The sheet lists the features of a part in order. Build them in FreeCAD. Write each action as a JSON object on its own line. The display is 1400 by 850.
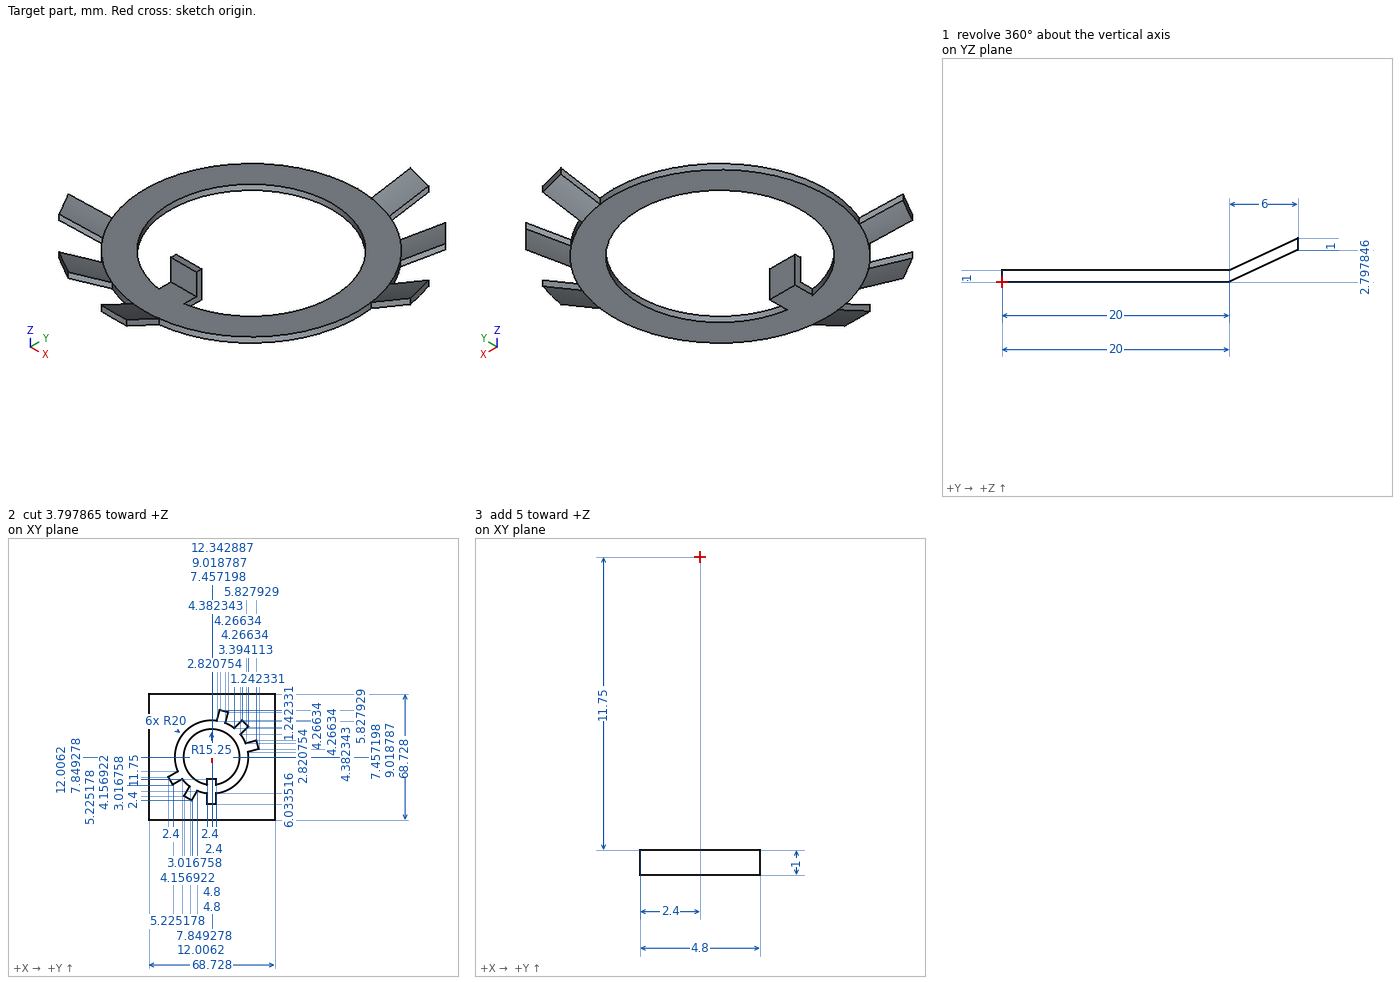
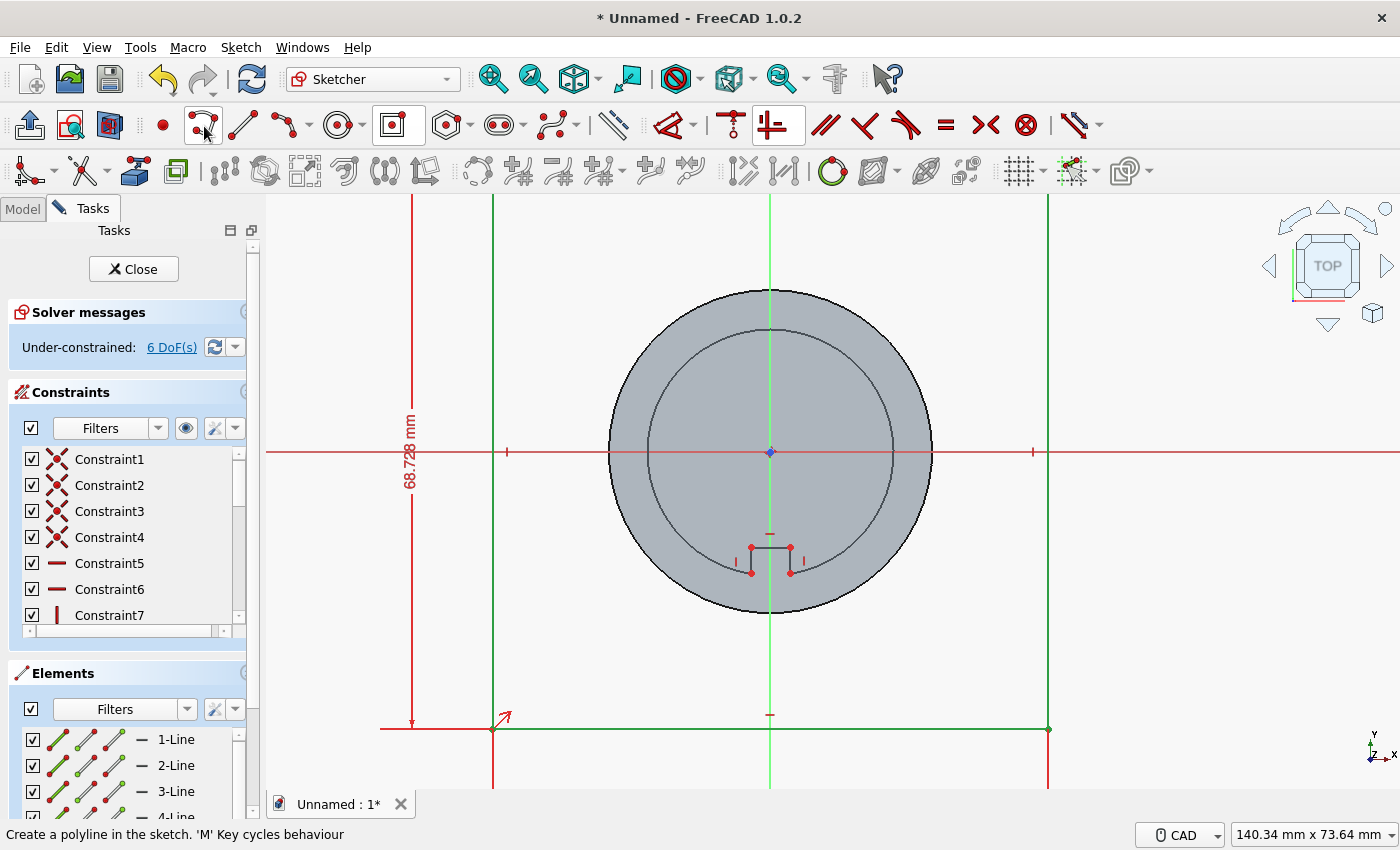
{"action": "left_click", "coordinate": [707, 600]}
{"action": "left_click", "coordinate": [683, 642]}
{"action": "left_click", "coordinate": [649, 623]}
{"action": "left_click", "coordinate": [673, 581]}
{"action": "right_click", "coordinate": [673, 581]}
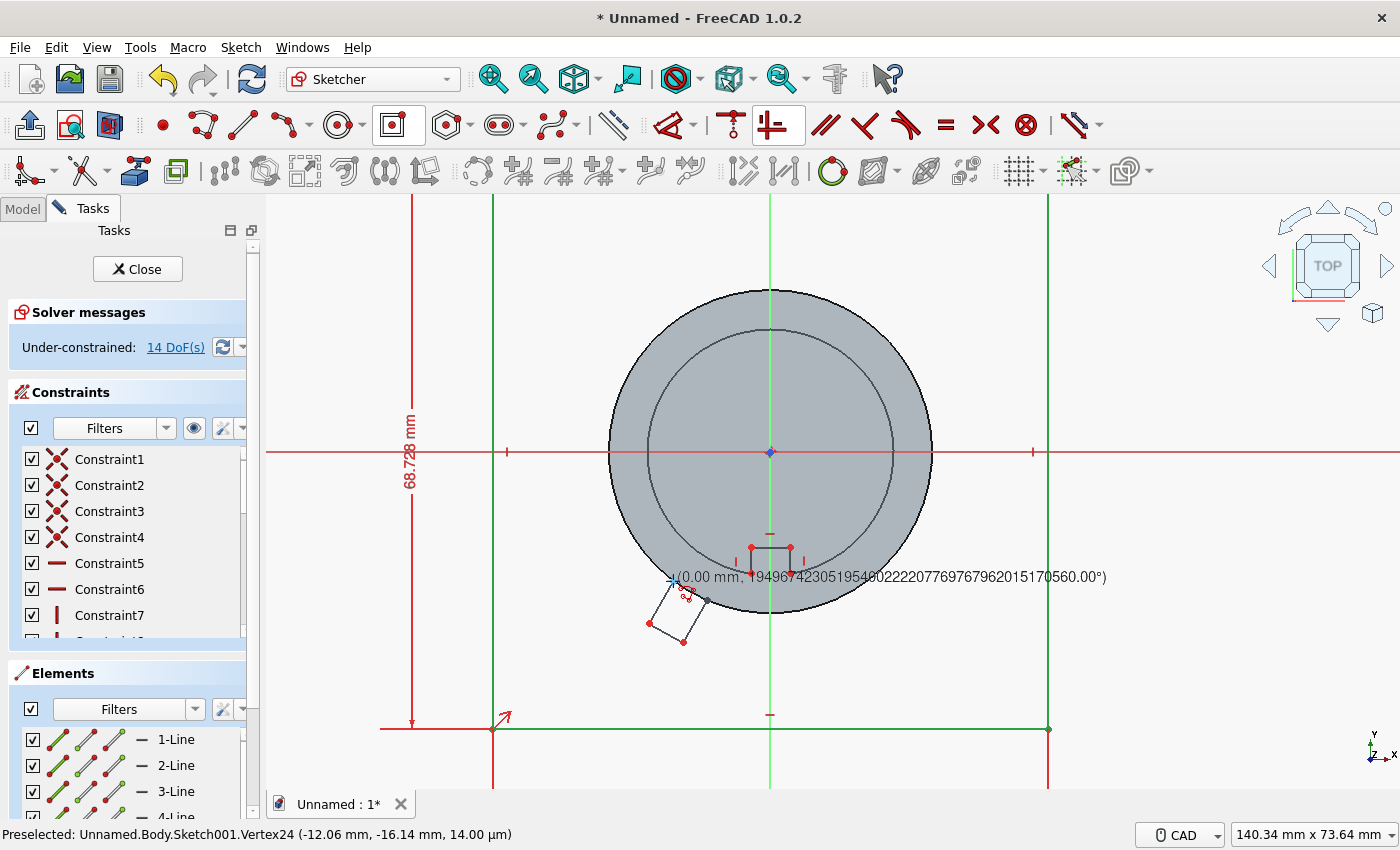
{"action": "left_click", "coordinate": [641, 549]}
{"action": "left_click", "coordinate": [599, 573]}
{"action": "left_click", "coordinate": [580, 539]}
{"action": "left_click", "coordinate": [622, 515]}
{"action": "right_click", "coordinate": [622, 515]}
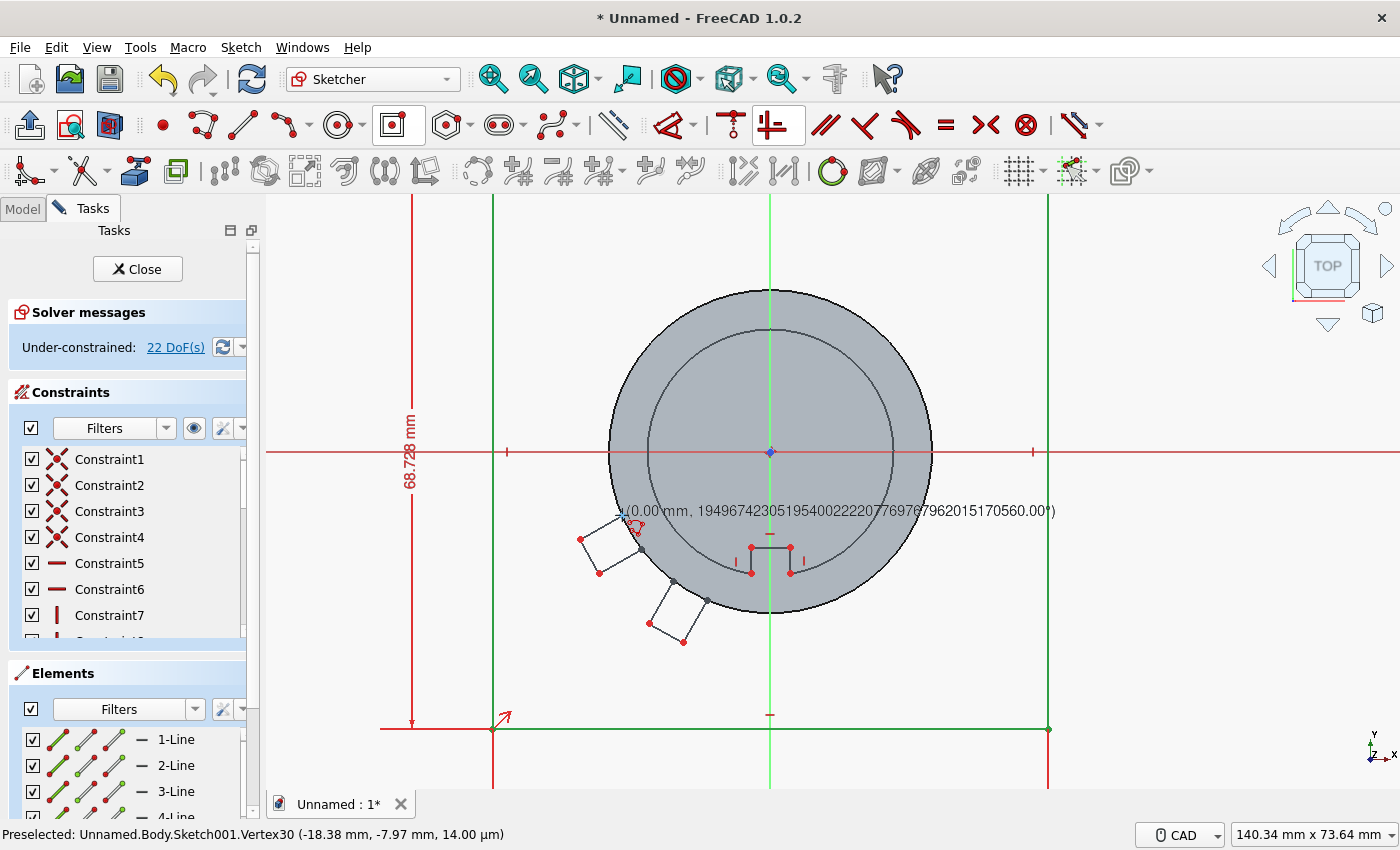
{"action": "left_click", "coordinate": [793, 292]}
{"action": "left_click", "coordinate": [806, 245]}
{"action": "left_click", "coordinate": [843, 255]}
{"action": "left_click", "coordinate": [831, 302]}
{"action": "right_click", "coordinate": [831, 302]}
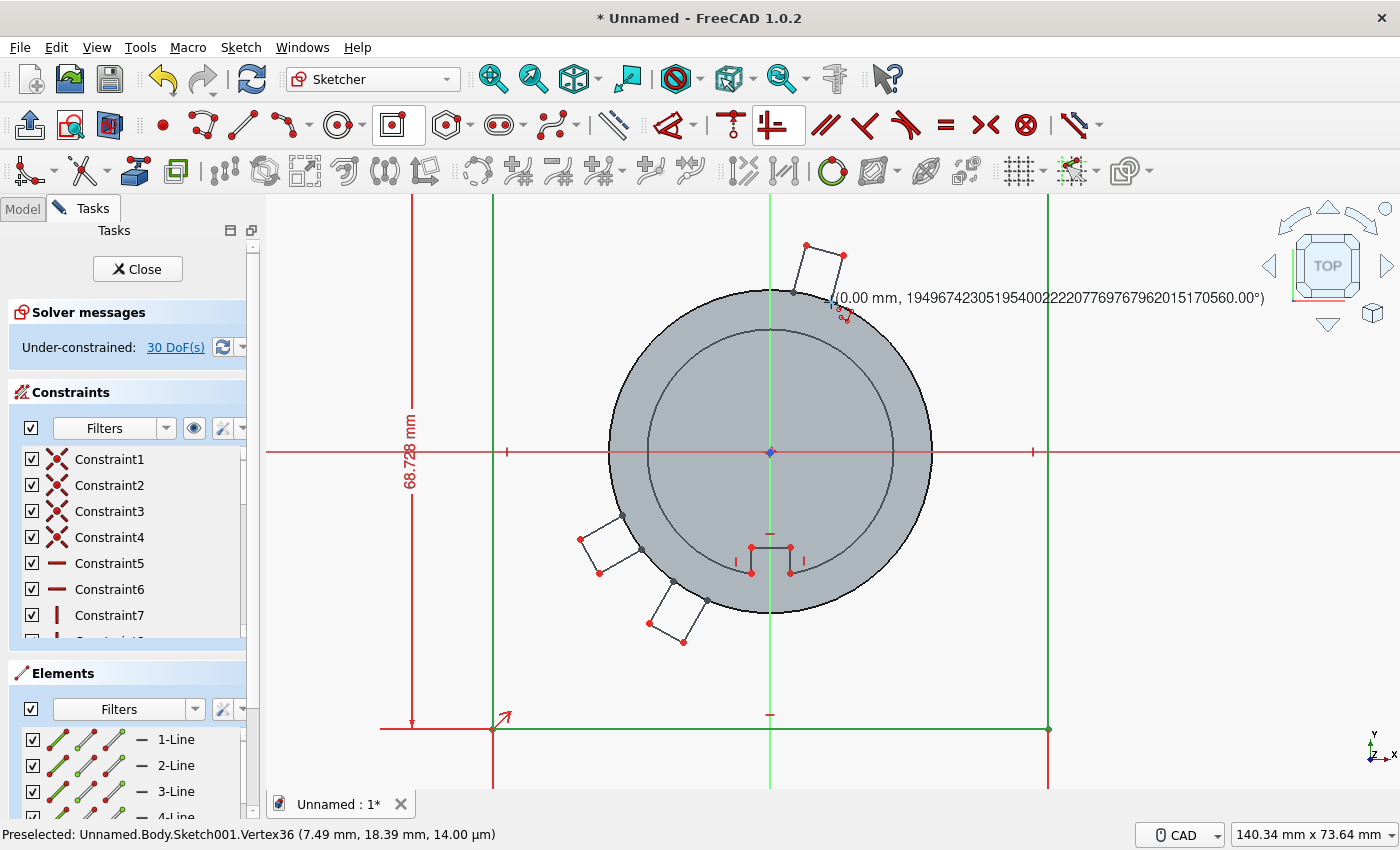
{"action": "left_click", "coordinate": [870, 324]}
{"action": "left_click", "coordinate": [905, 290]}
{"action": "left_click", "coordinate": [932, 317]}
{"action": "left_click", "coordinate": [898, 352]}
{"action": "right_click", "coordinate": [898, 352]}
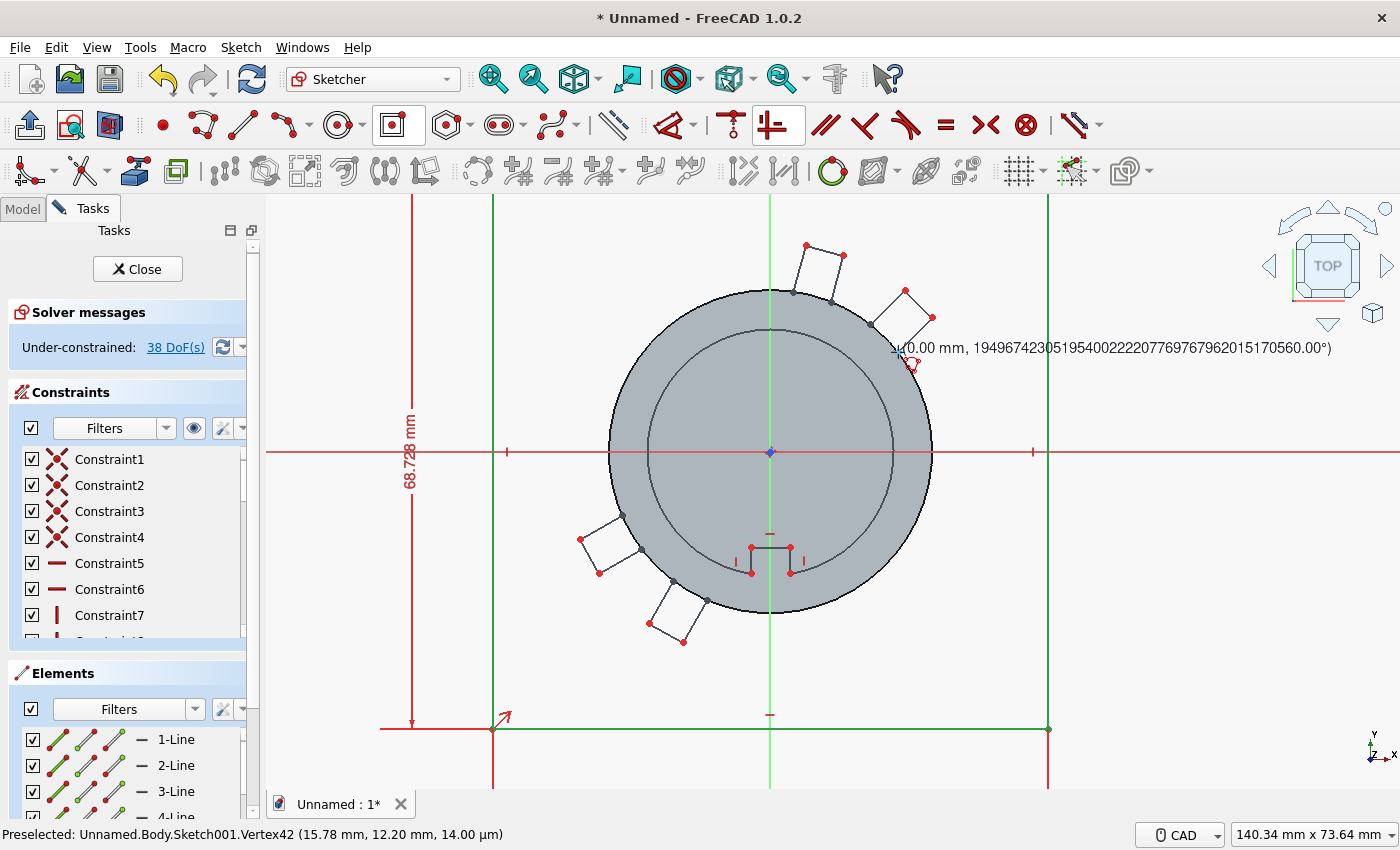
{"action": "left_click", "coordinate": [920, 391]}
{"action": "left_click", "coordinate": [968, 379]}
{"action": "left_click", "coordinate": [978, 416]}
{"action": "left_click", "coordinate": [930, 429]}
{"action": "right_click", "coordinate": [930, 429]}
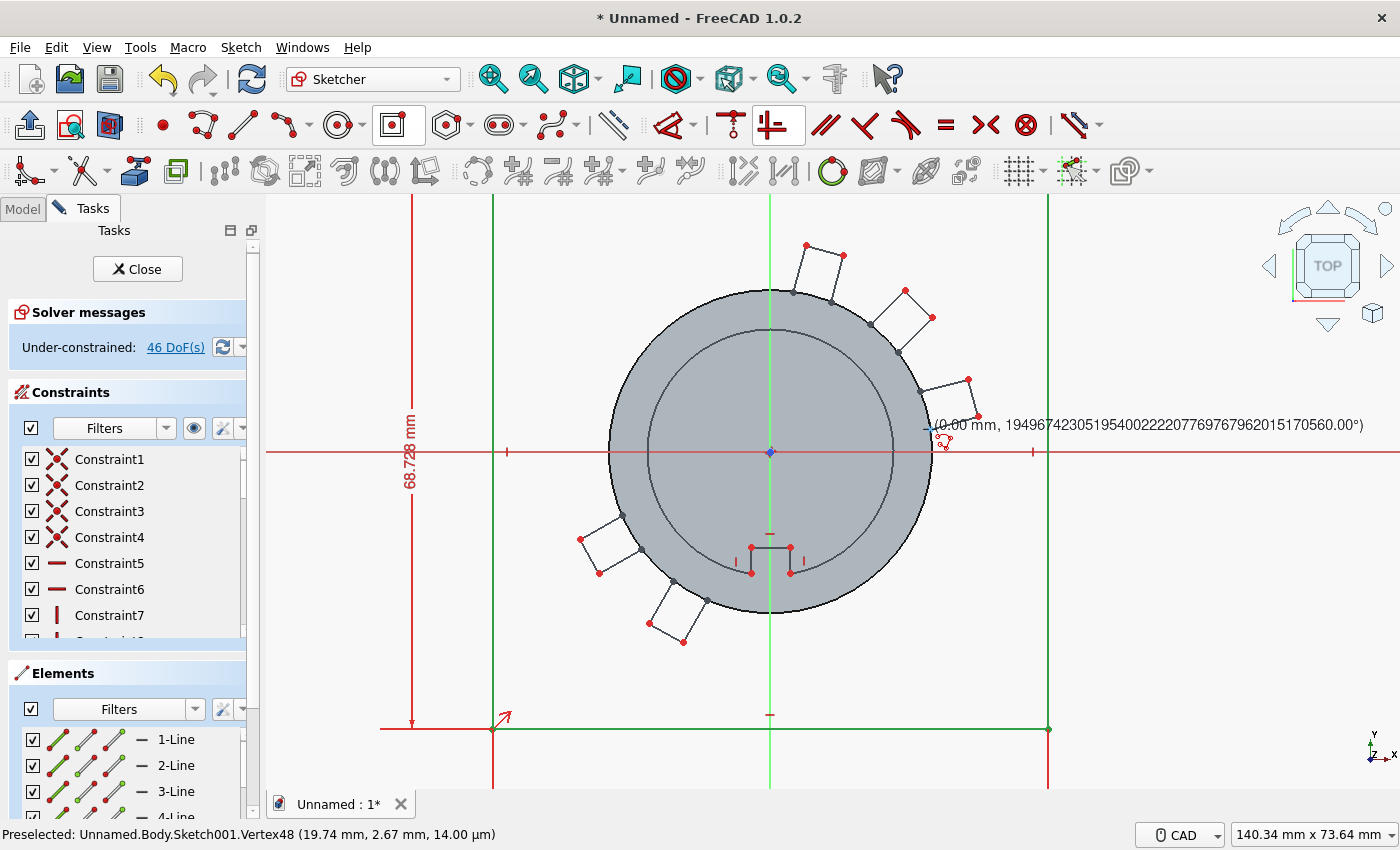
{"action": "left_click", "coordinate": [790, 612]}
{"action": "left_click", "coordinate": [790, 661]}
{"action": "left_click", "coordinate": [751, 661]}
{"action": "left_click", "coordinate": [751, 612]}
{"action": "right_click", "coordinate": [751, 612]}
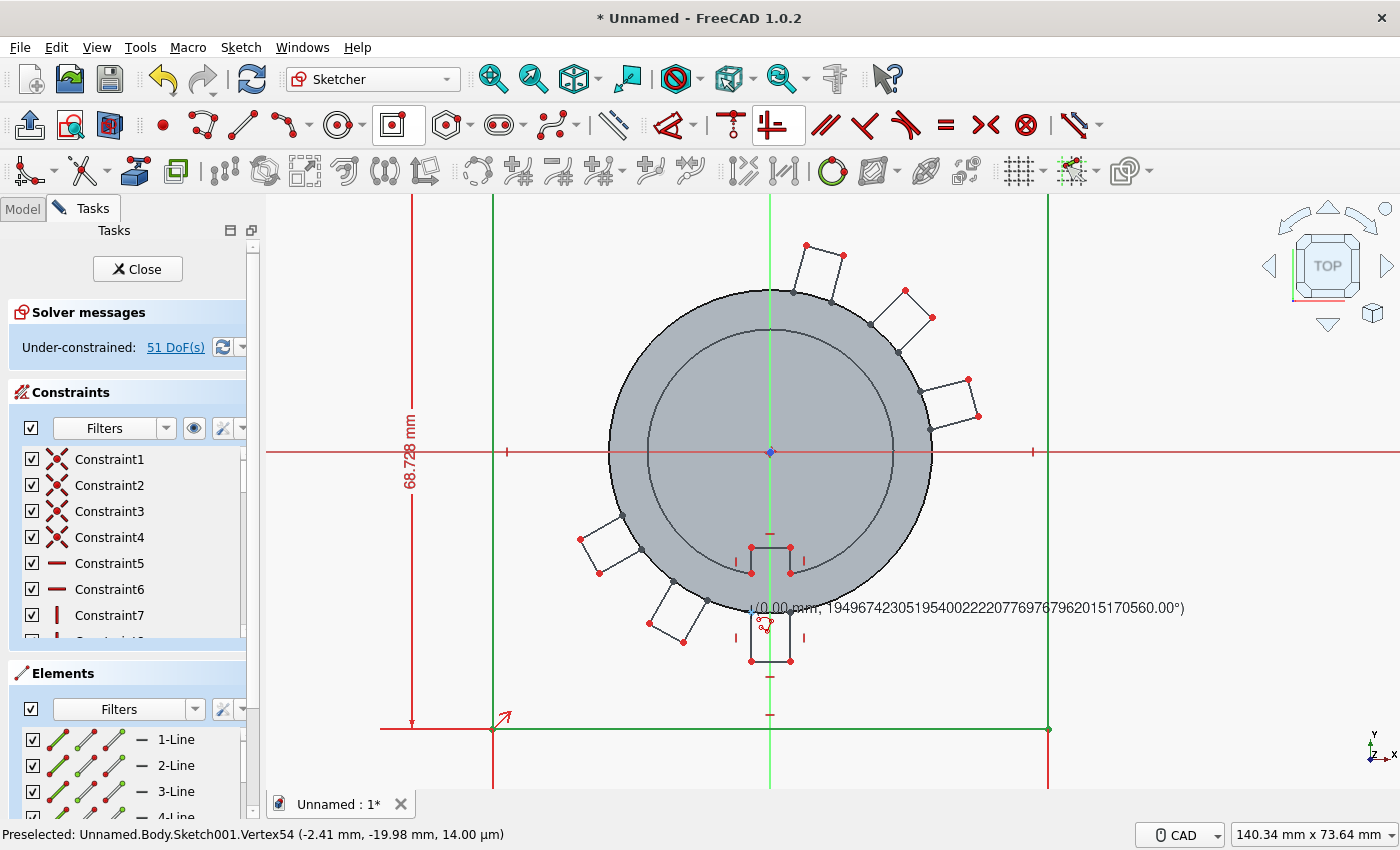
{"action": "left_click", "coordinate": [284, 126]}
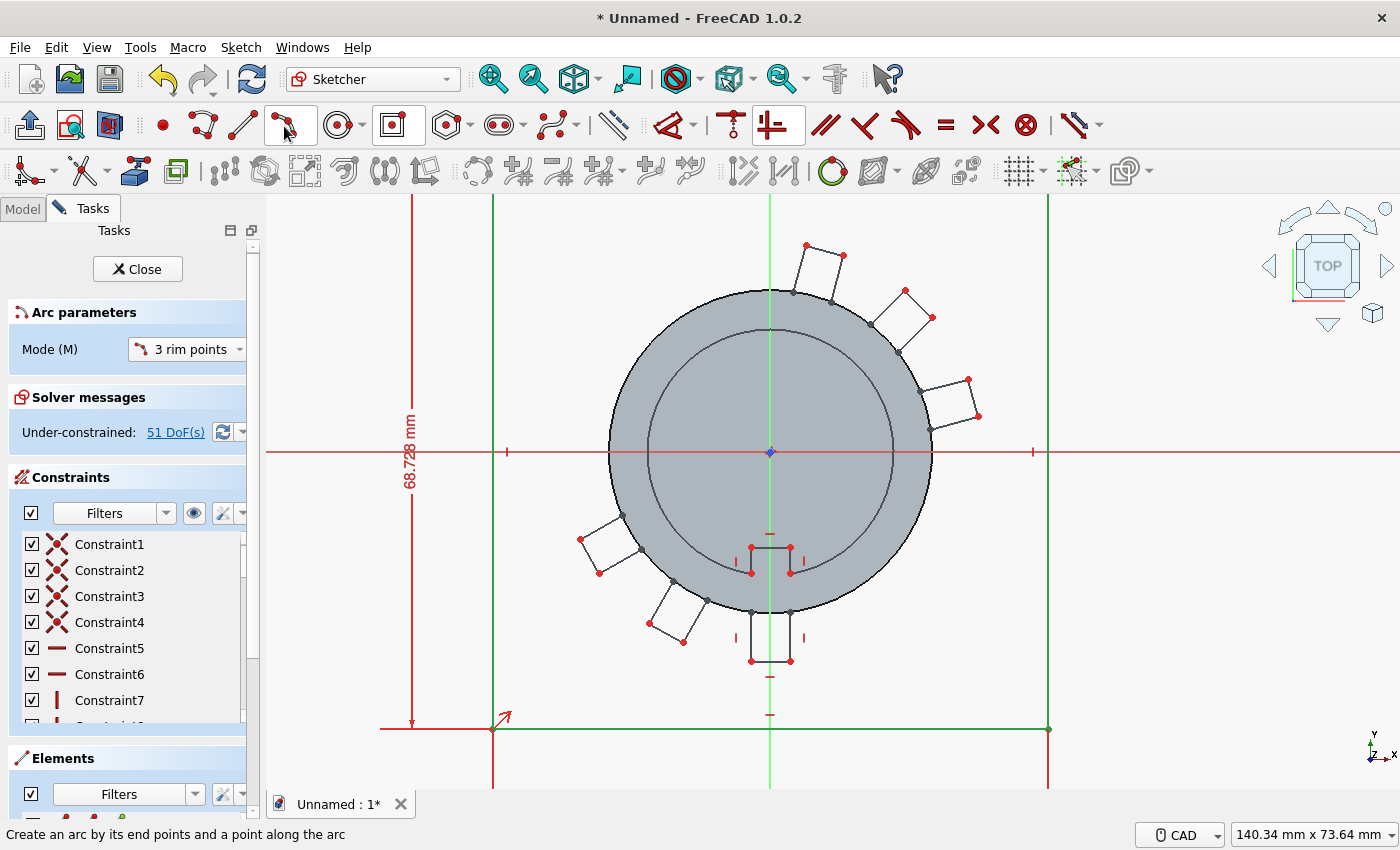
{"action": "left_click", "coordinate": [673, 582]}
{"action": "left_click", "coordinate": [641, 550]}